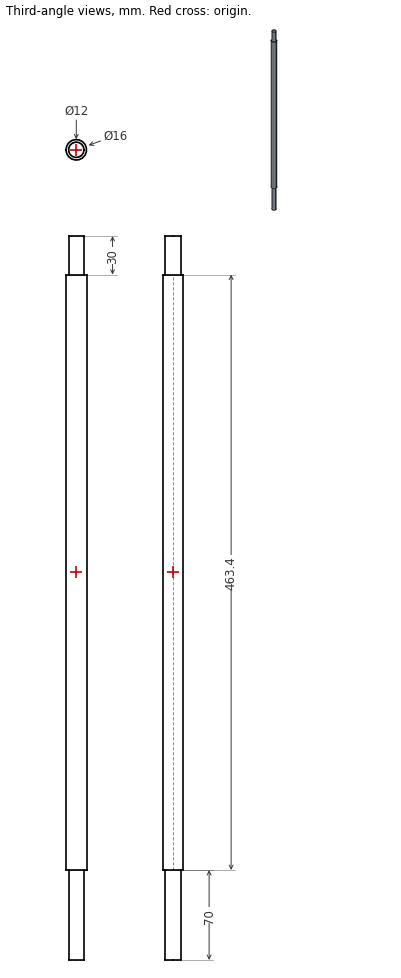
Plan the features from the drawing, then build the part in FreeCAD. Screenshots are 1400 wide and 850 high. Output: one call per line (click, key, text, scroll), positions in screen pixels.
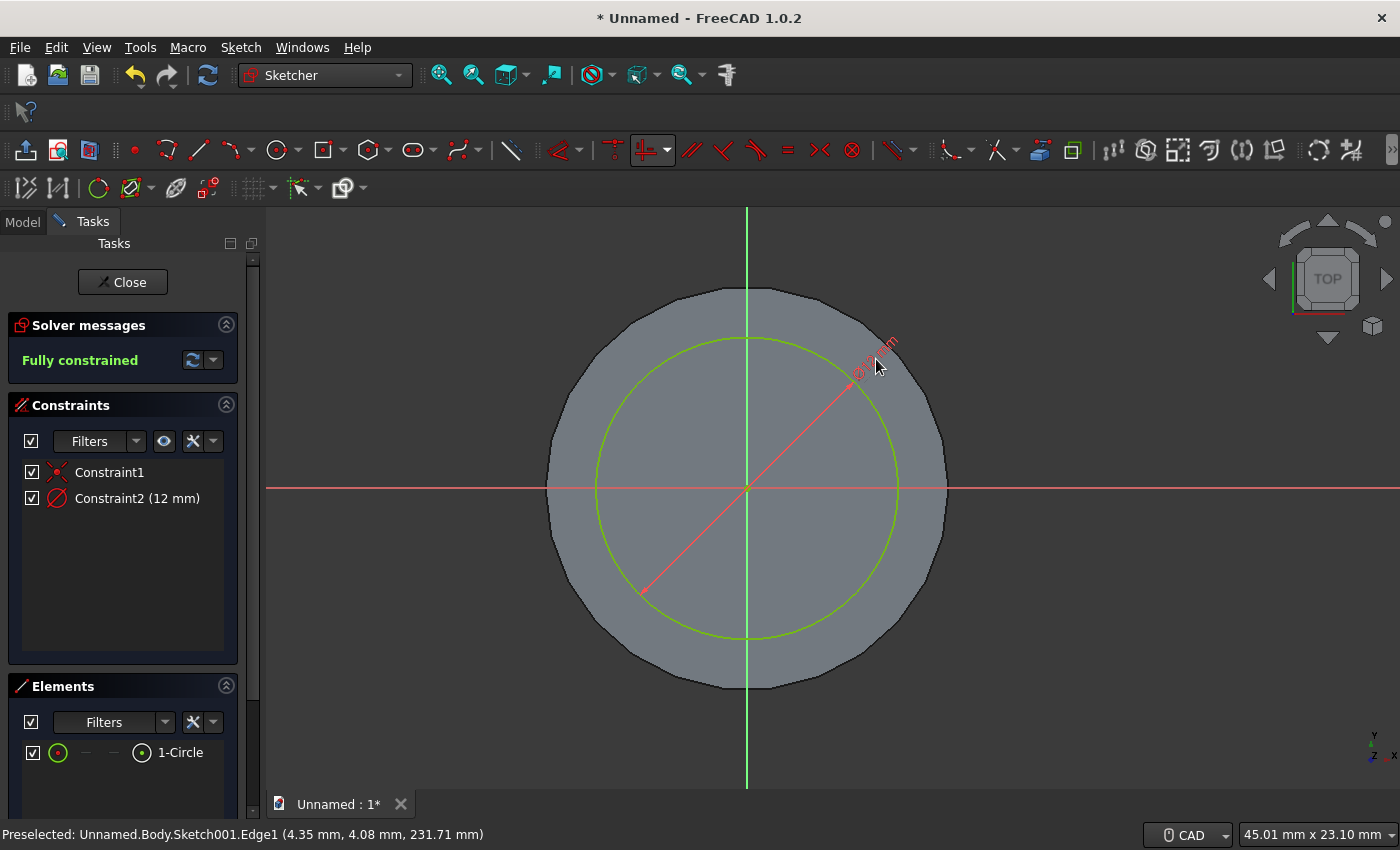
click(123, 282)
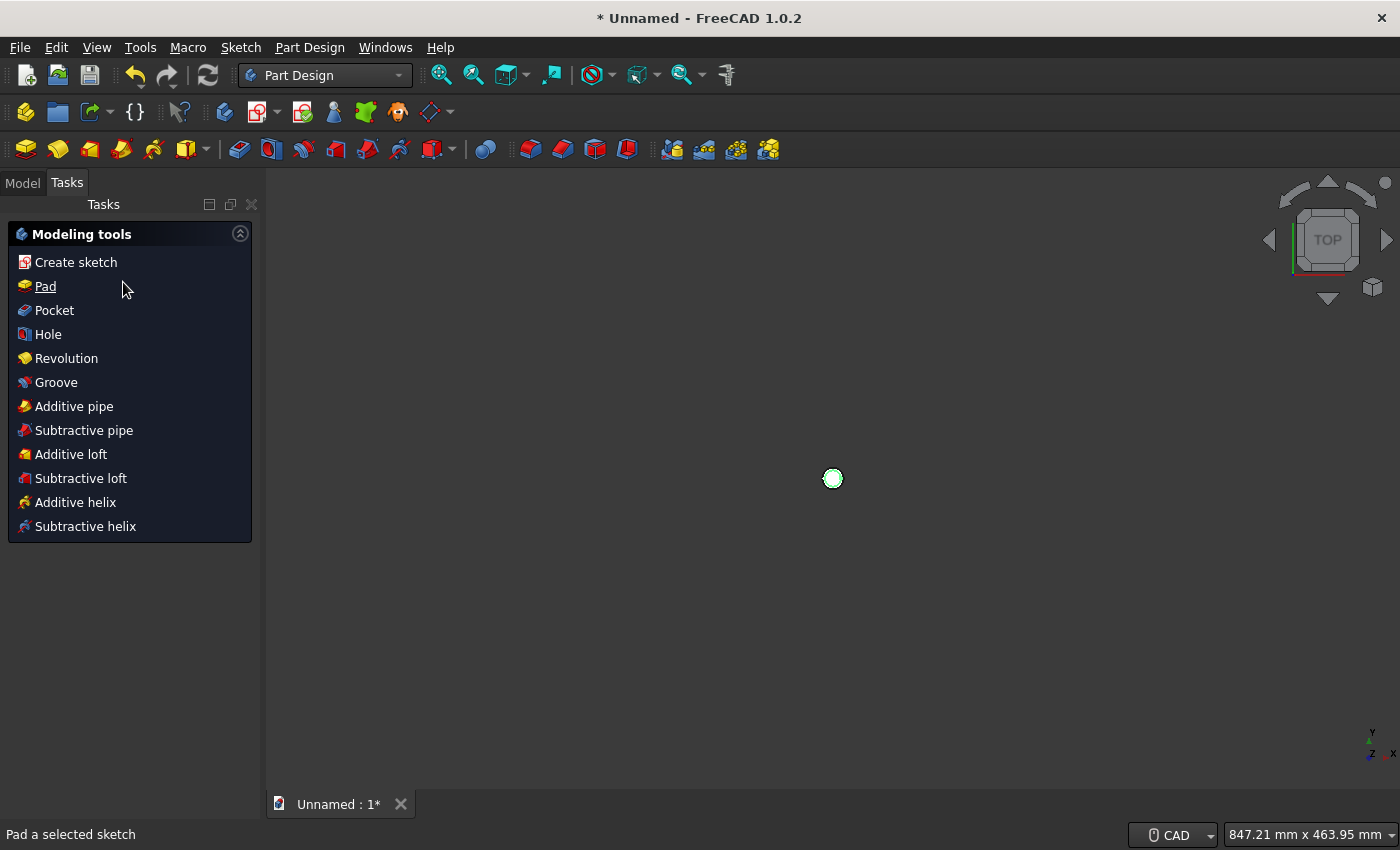
click(26, 150)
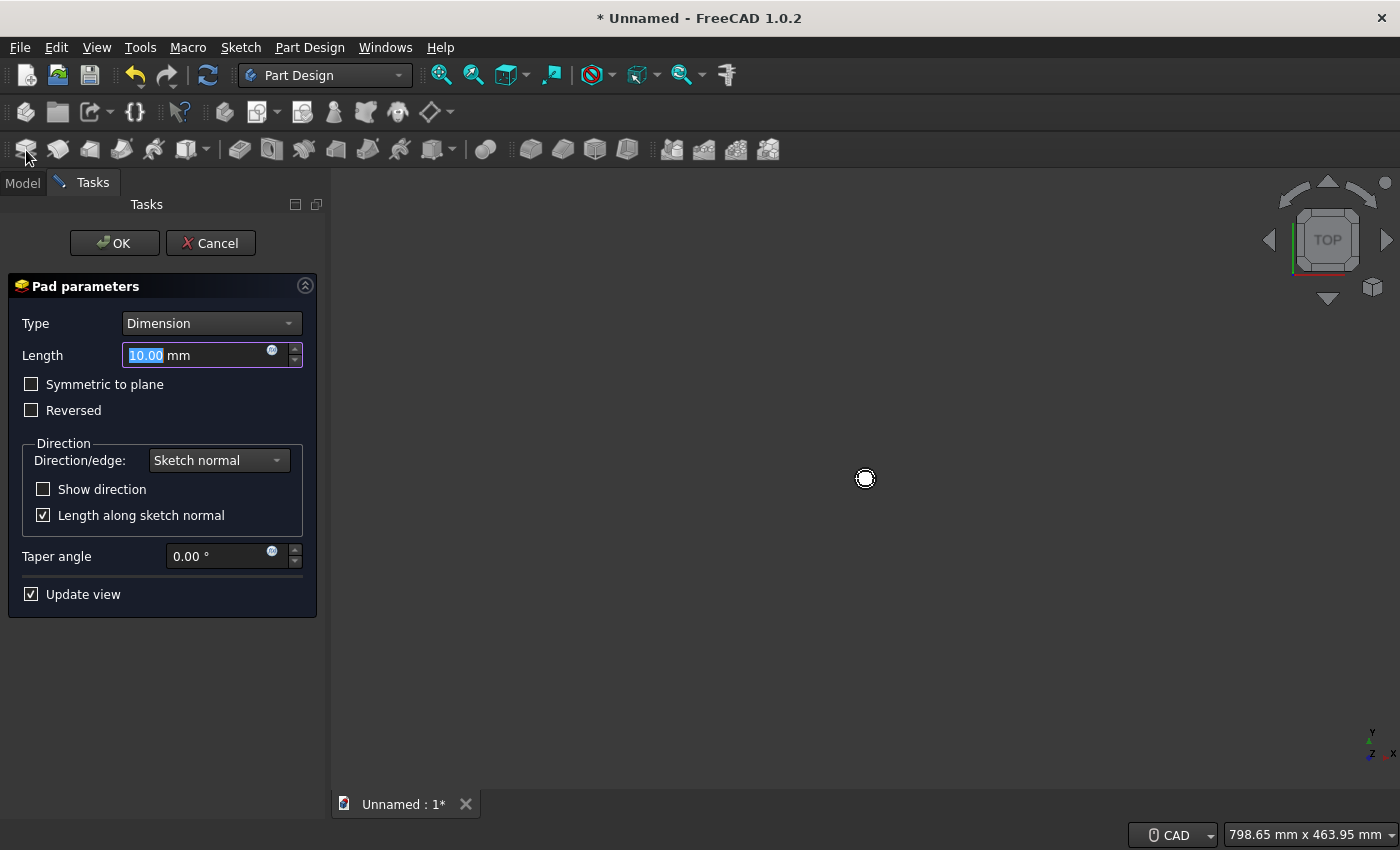
text(30)
key(Tab)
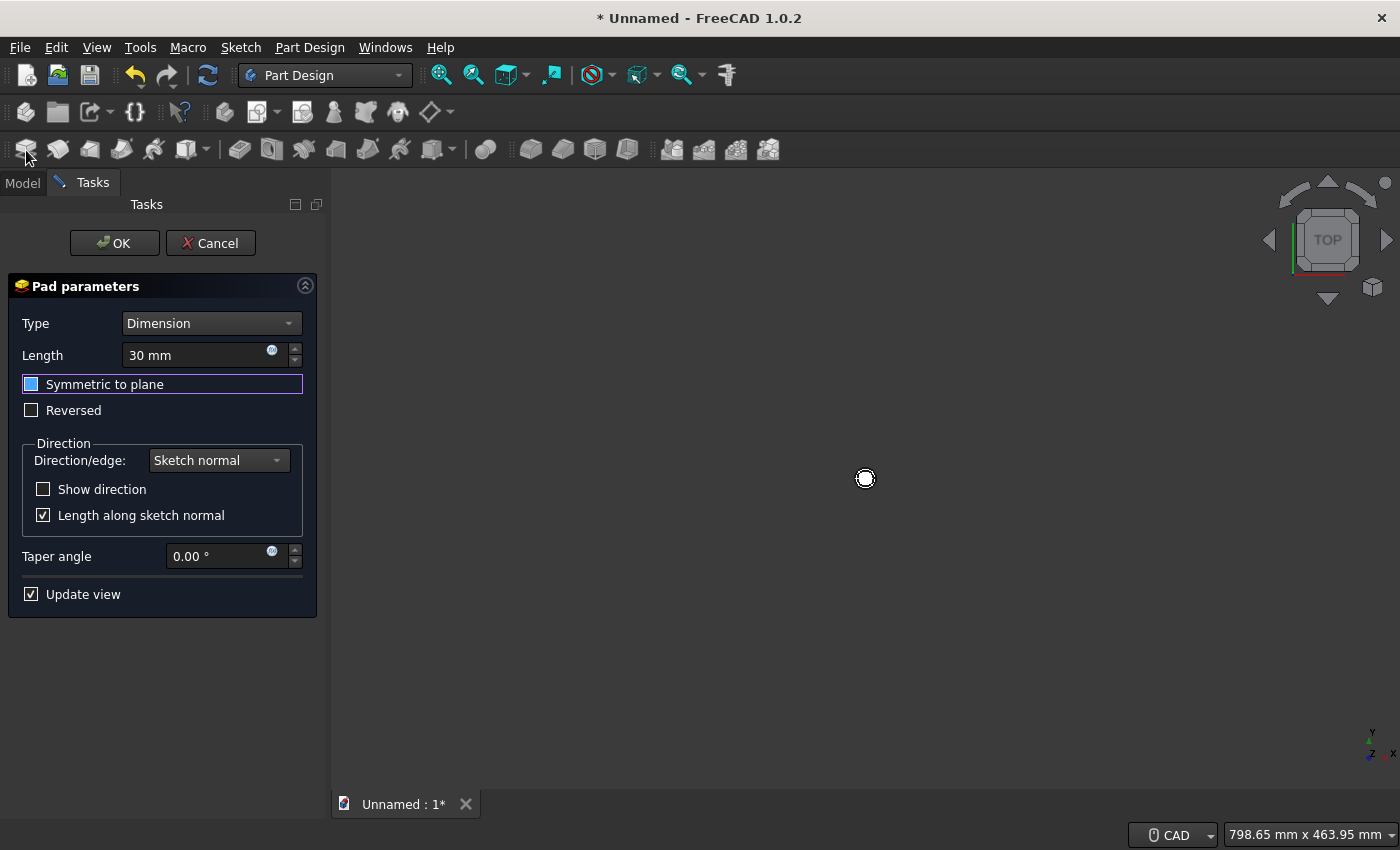
click(115, 243)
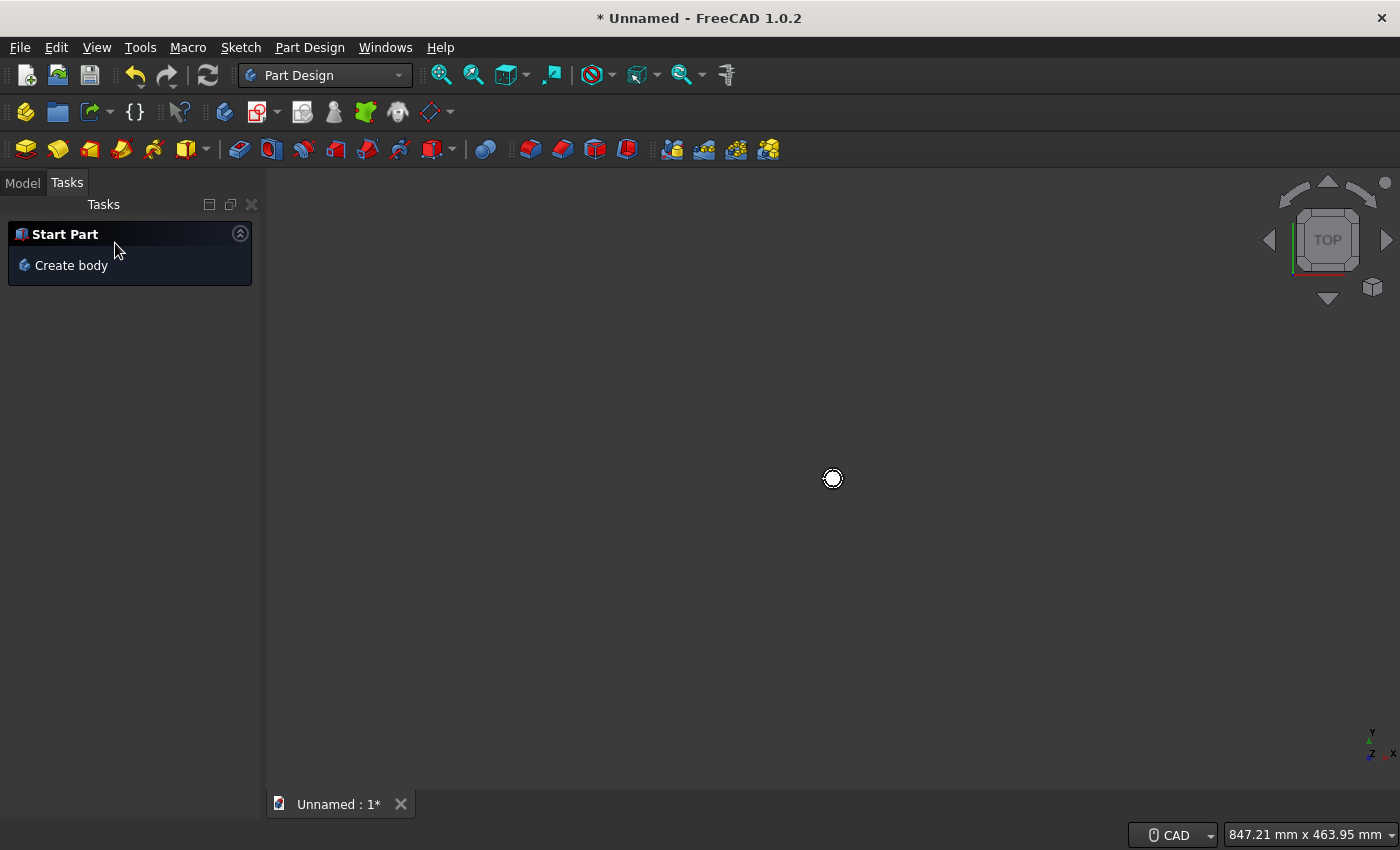
click(442, 76)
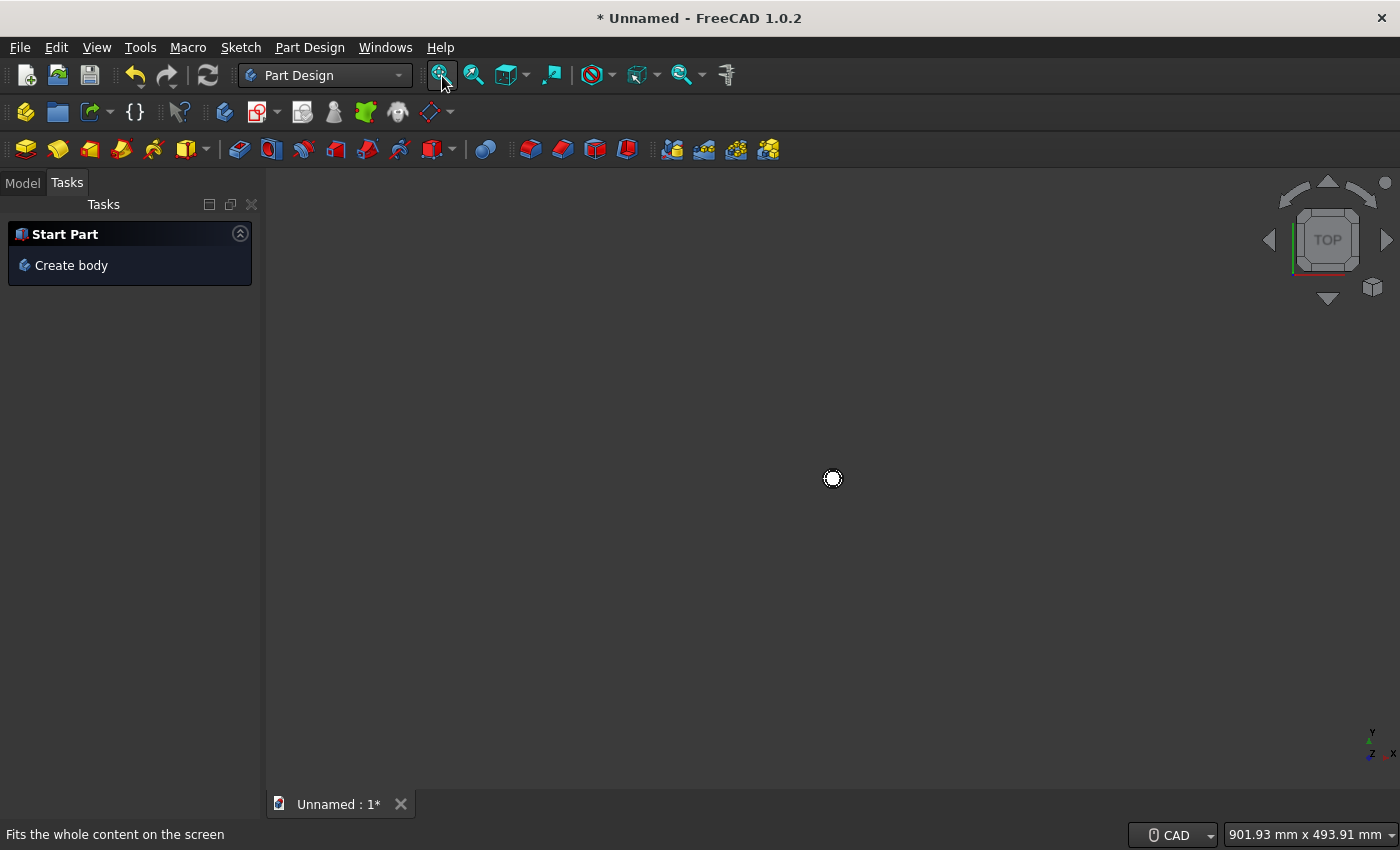
click(23, 182)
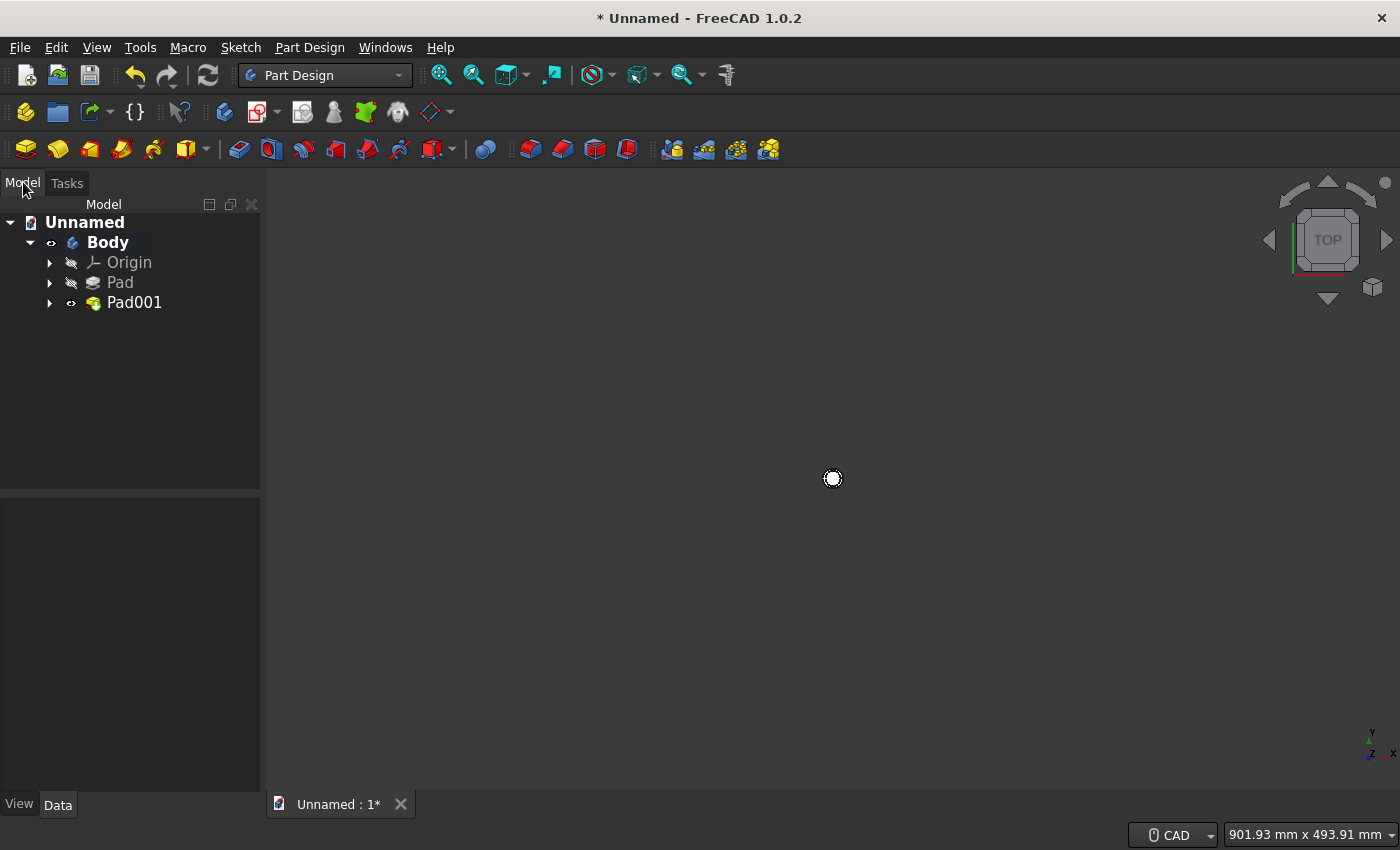
click(50, 263)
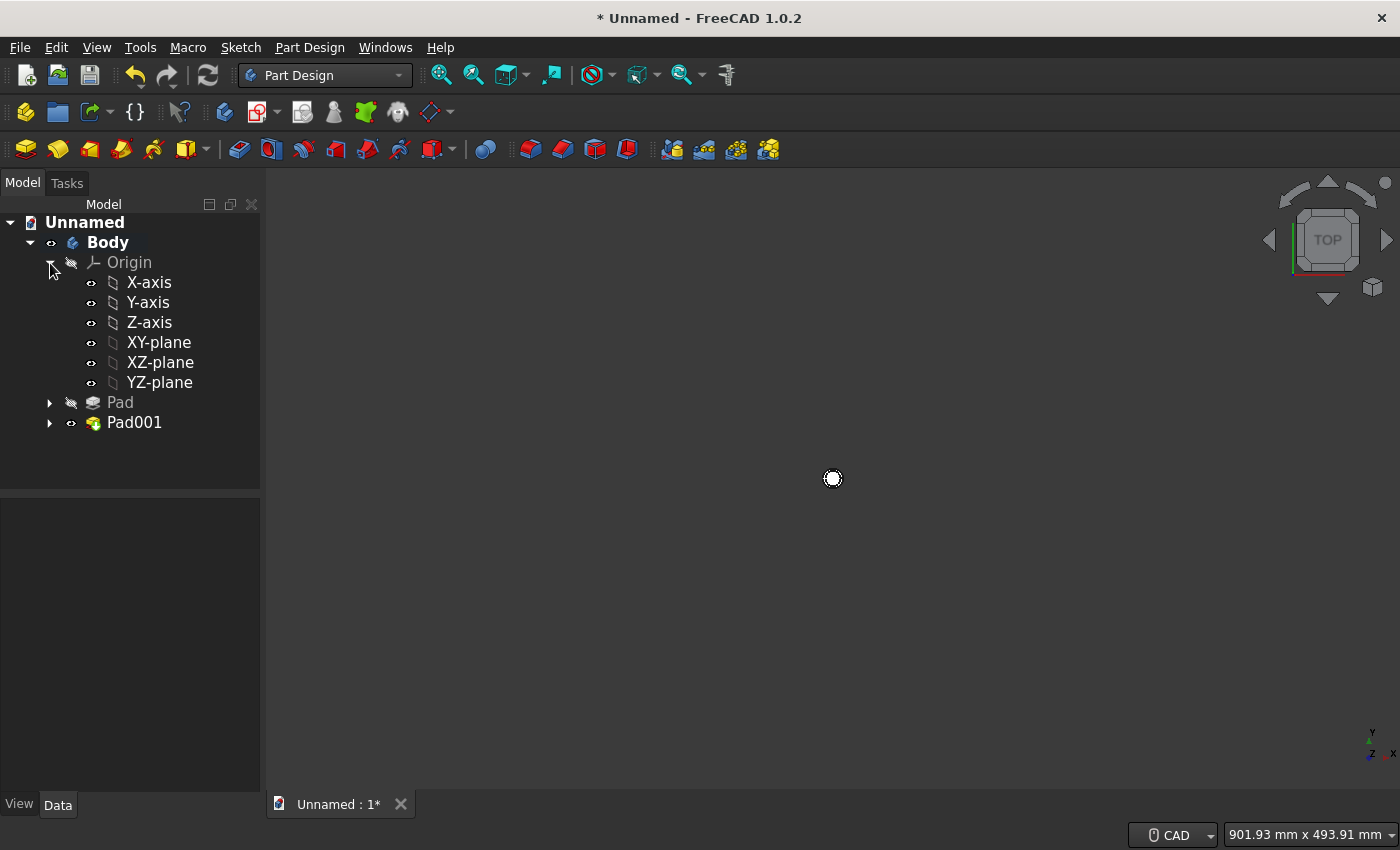
click(136, 343)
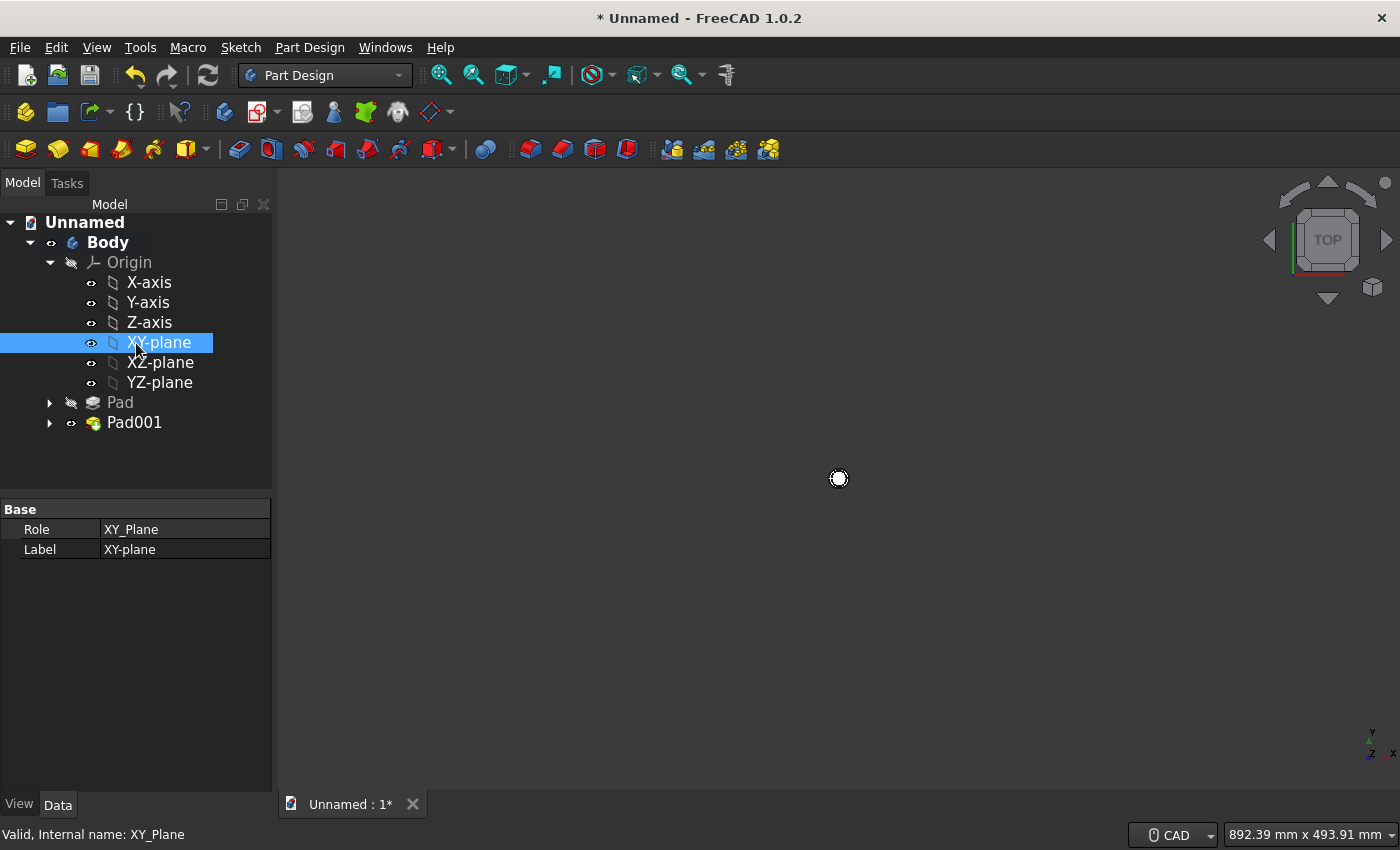
click(430, 112)